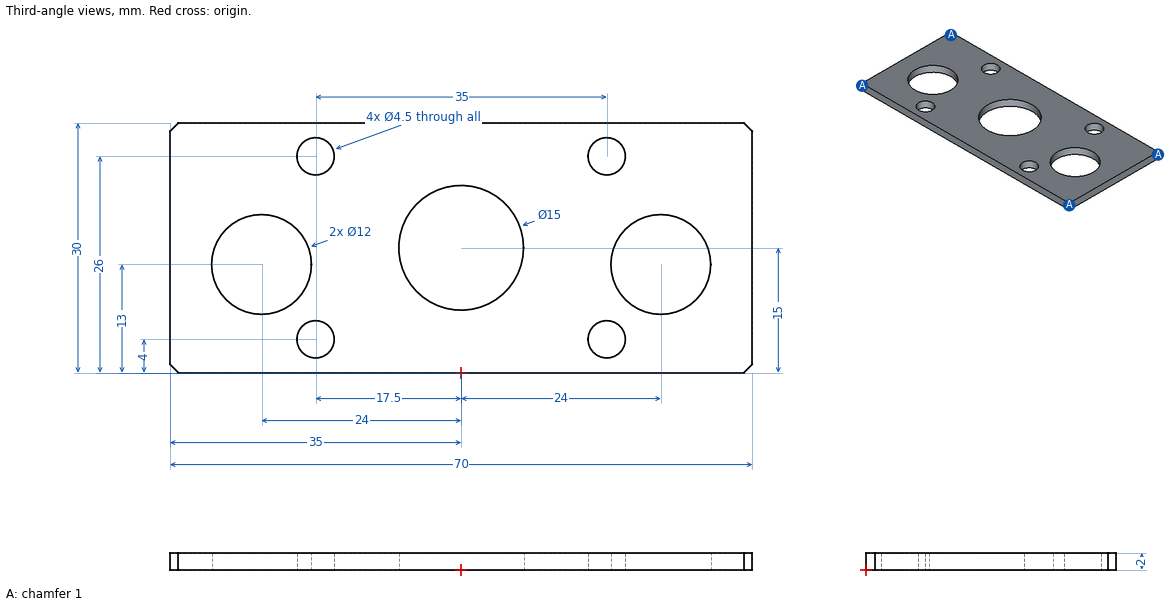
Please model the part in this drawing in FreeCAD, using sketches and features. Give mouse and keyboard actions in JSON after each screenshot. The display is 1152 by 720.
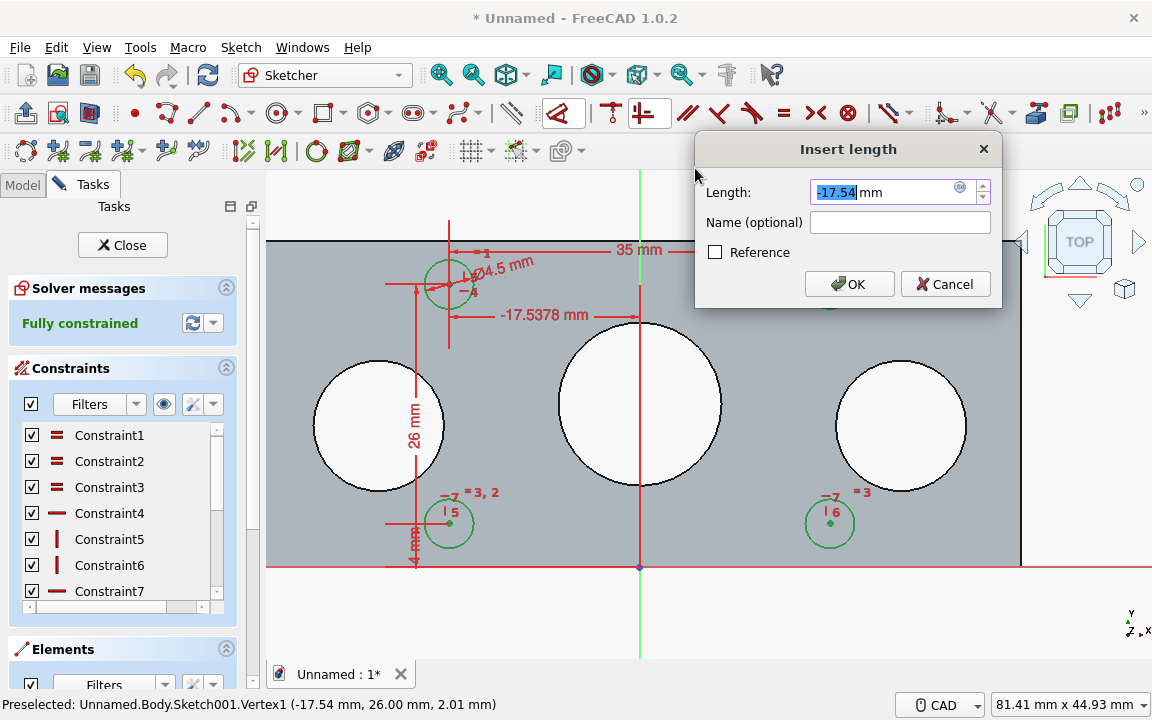
{"action": "type", "text": "-17.5"}
{"action": "key", "text": "Return"}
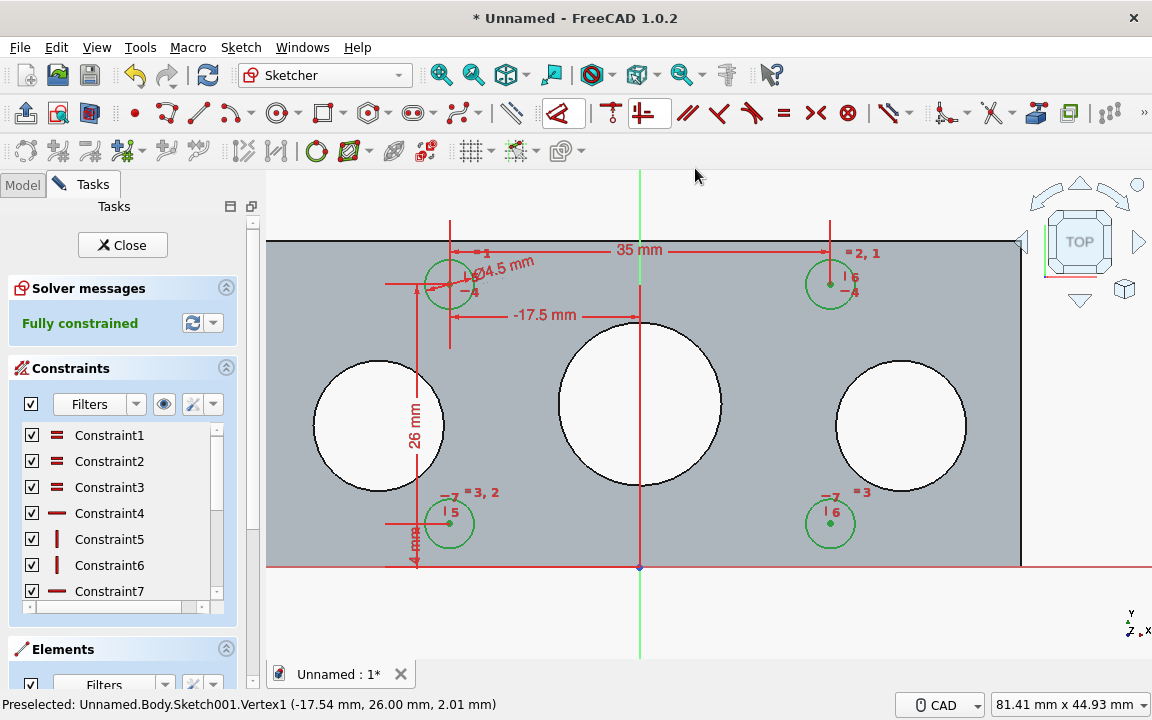
{"action": "left_click", "coordinate": [123, 245]}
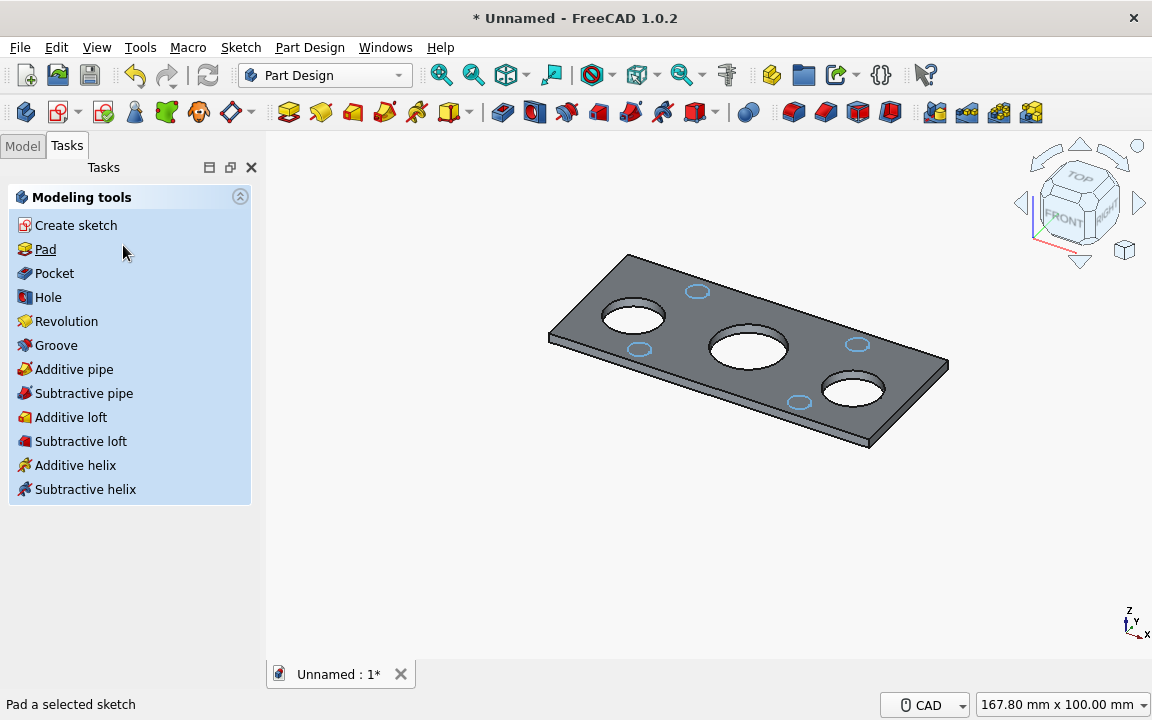
{"action": "left_click", "coordinate": [536, 112]}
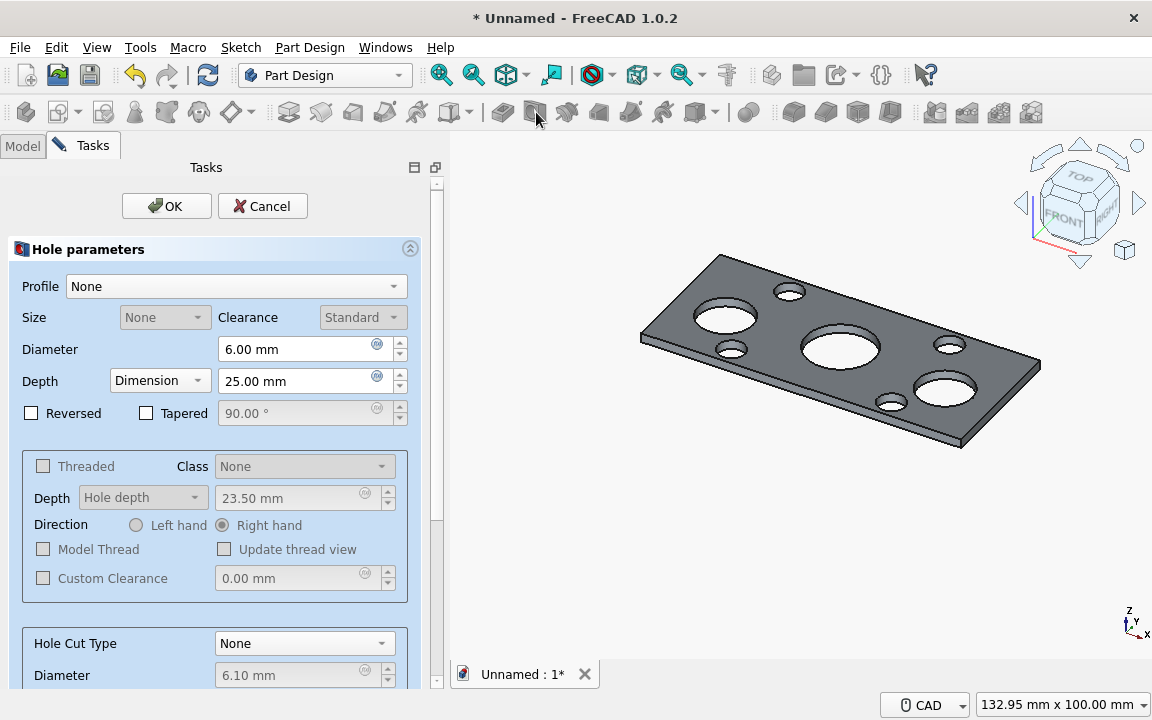
{"action": "triple_click", "coordinate": [305, 349]}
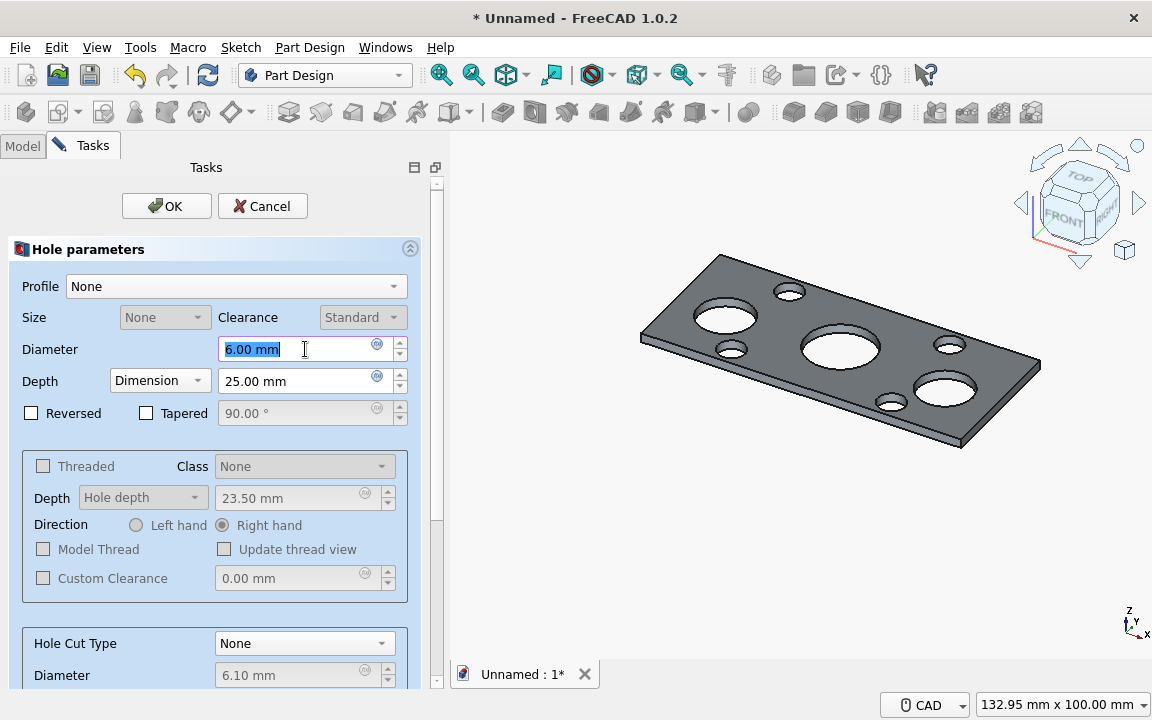
{"action": "type", "text": "4.5"}
{"action": "key", "text": "Tab"}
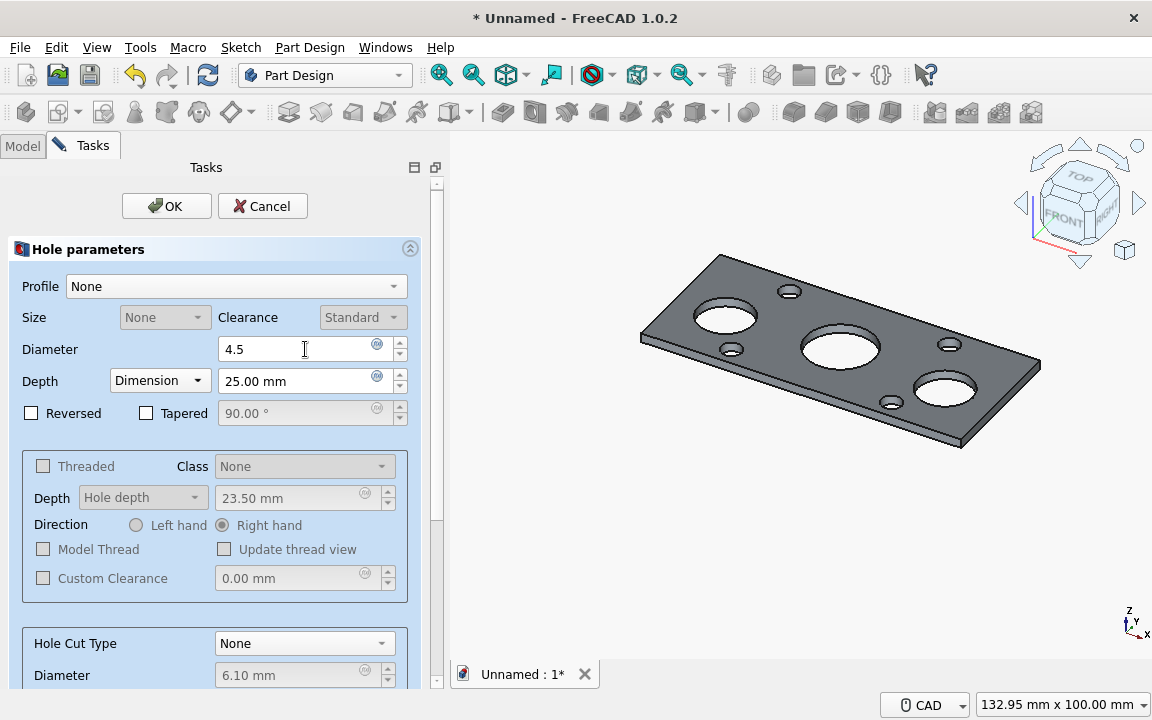
{"action": "left_click", "coordinate": [161, 380]}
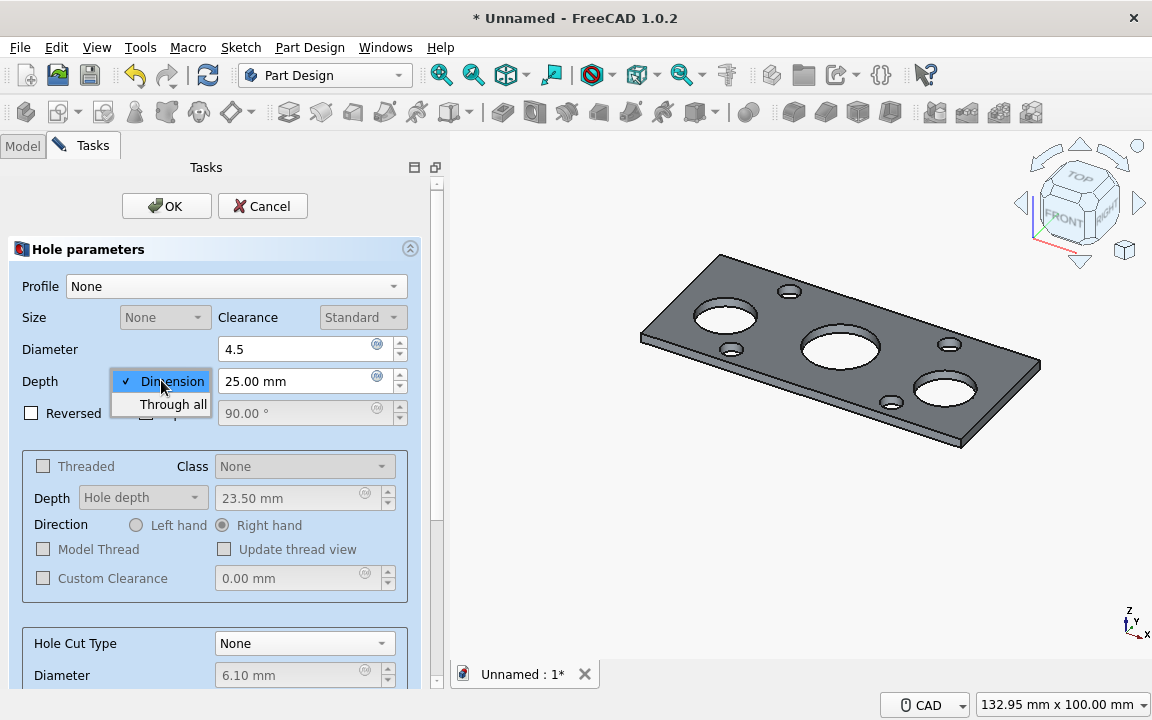
{"action": "left_click", "coordinate": [160, 404]}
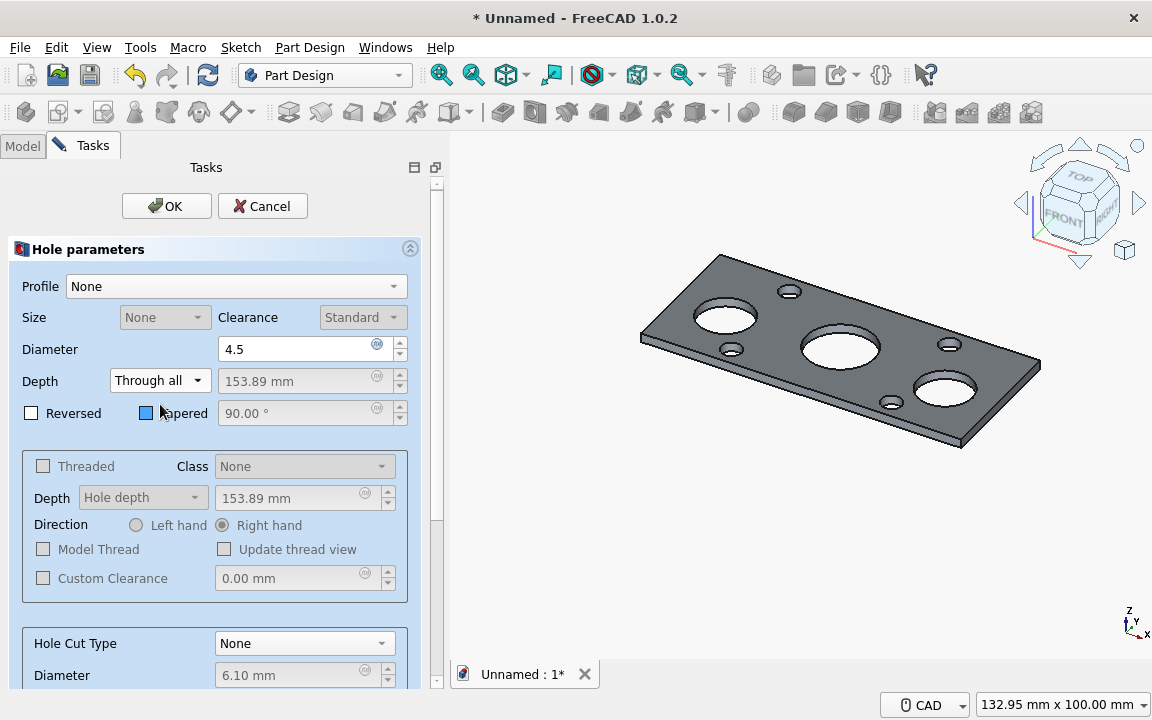
{"action": "left_click", "coordinate": [167, 206]}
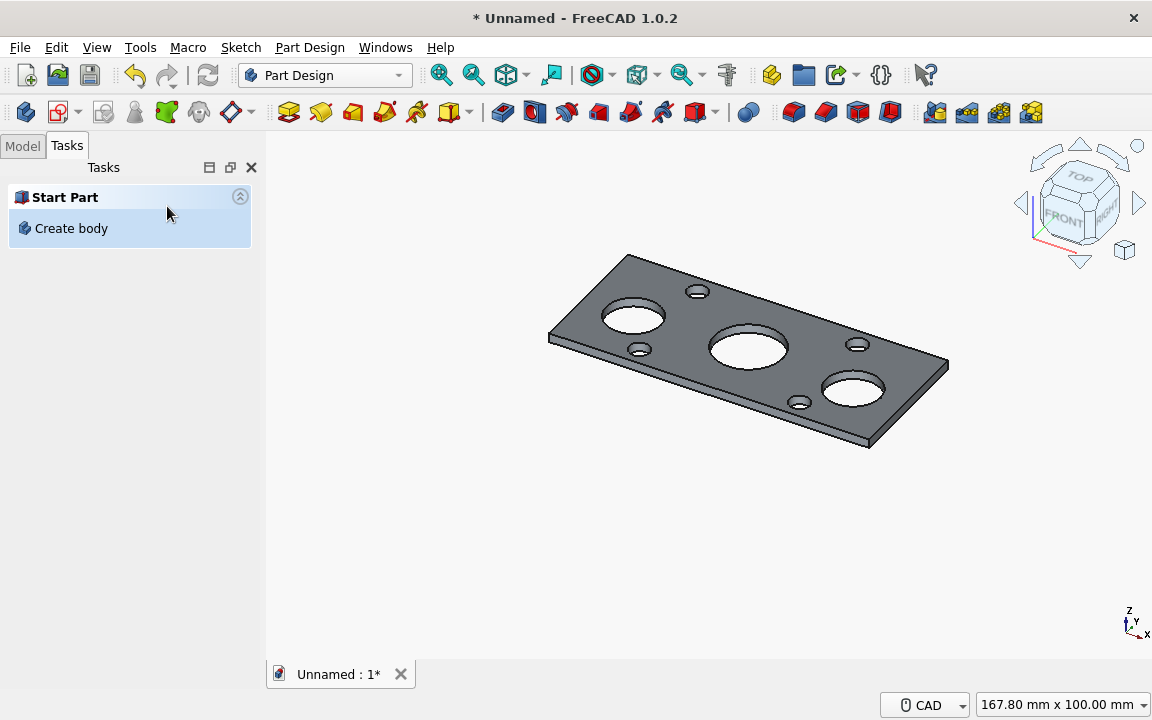
{"action": "left_click", "coordinate": [869, 445]}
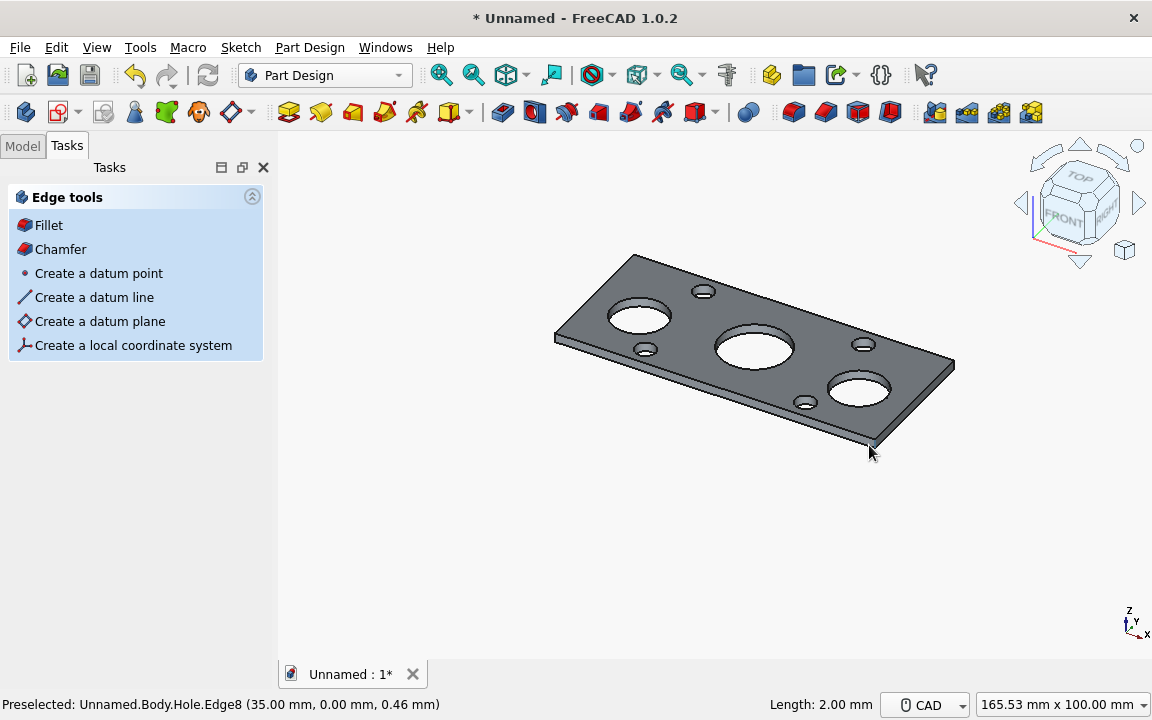
{"action": "scroll", "coordinate": [555, 337], "scroll_direction": "up", "scroll_amount": 7}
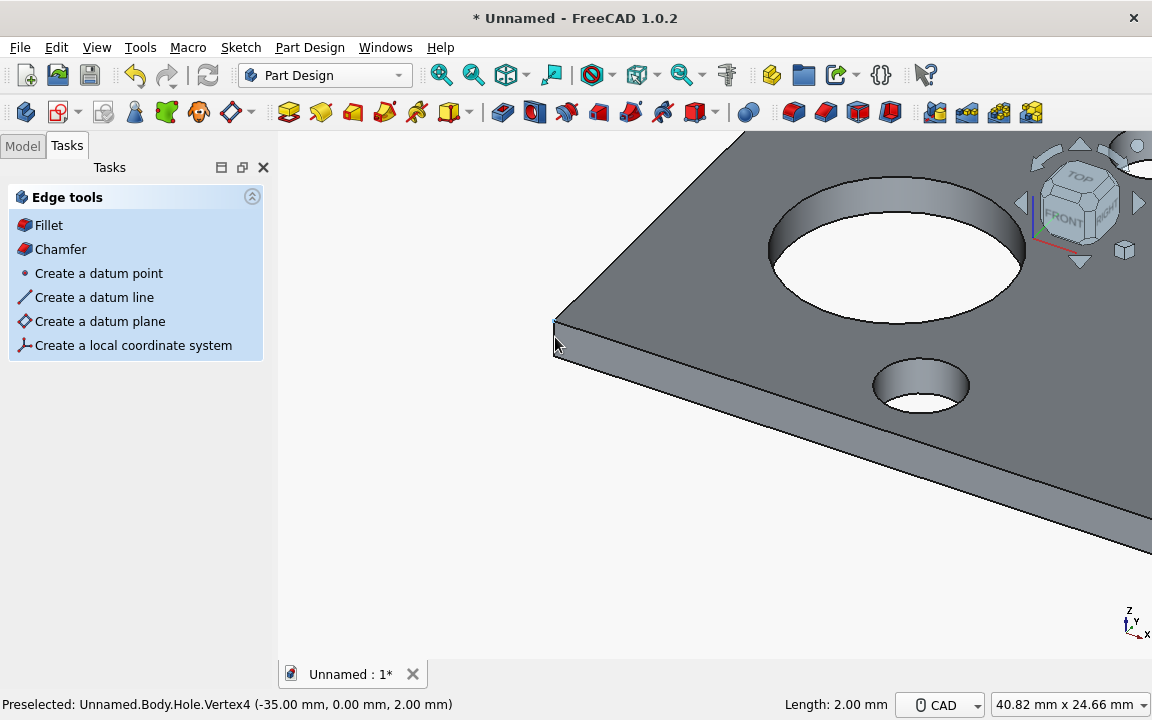
{"action": "left_click", "coordinate": [442, 76]}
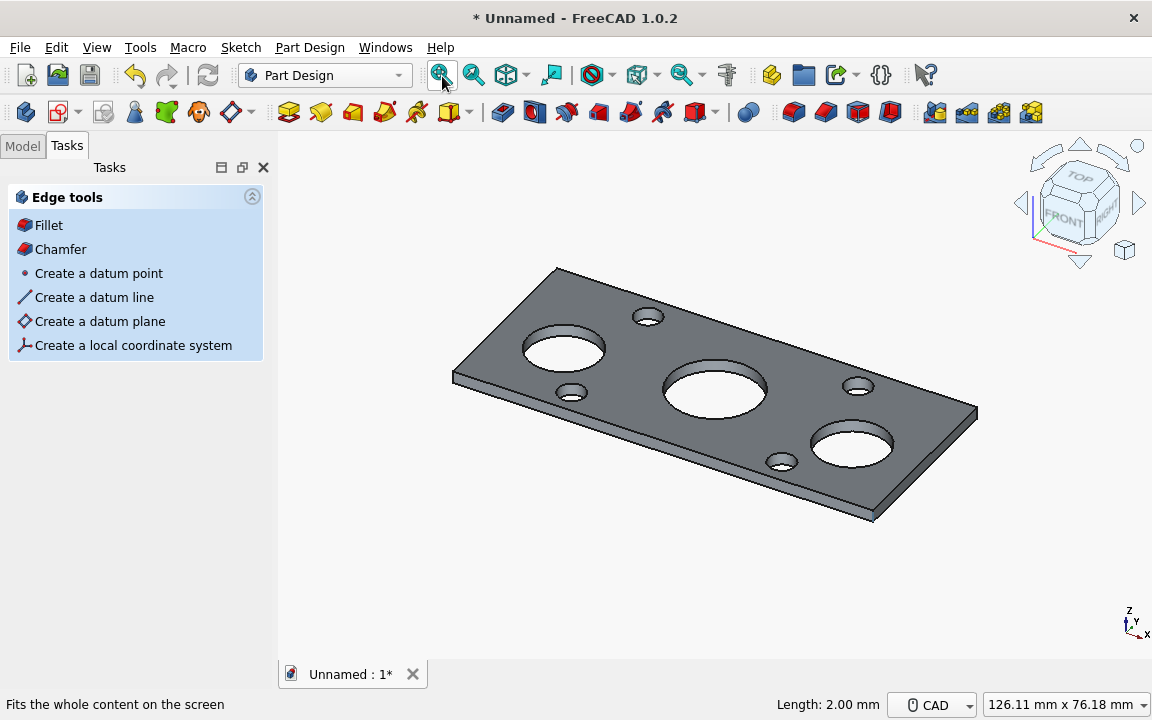
{"action": "key", "text": "0"}